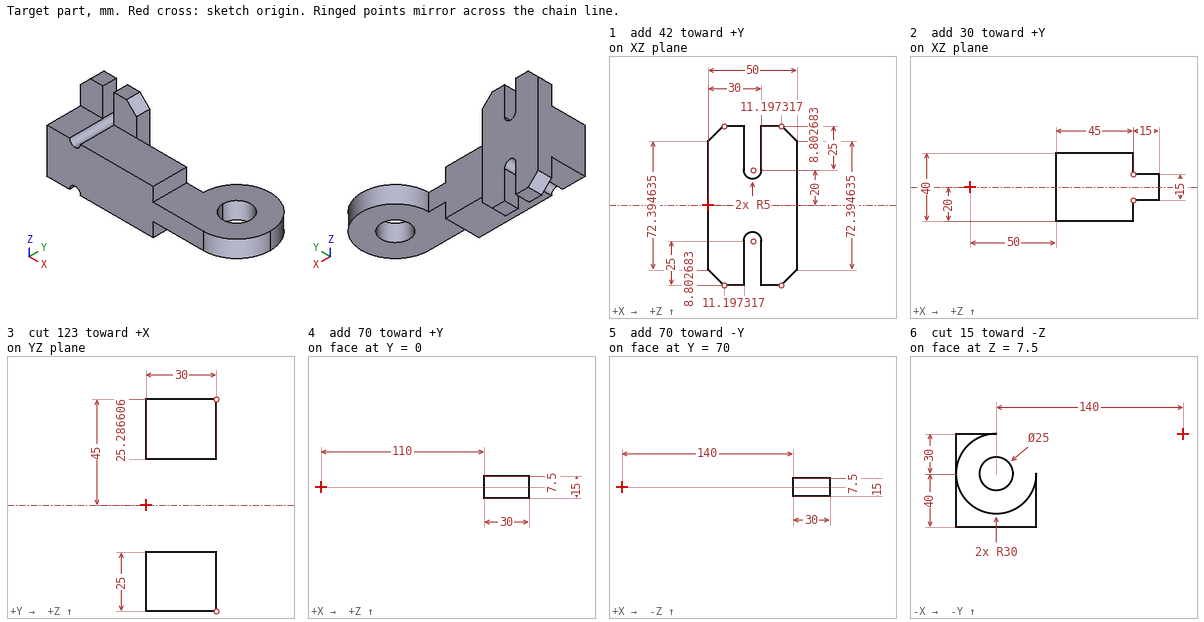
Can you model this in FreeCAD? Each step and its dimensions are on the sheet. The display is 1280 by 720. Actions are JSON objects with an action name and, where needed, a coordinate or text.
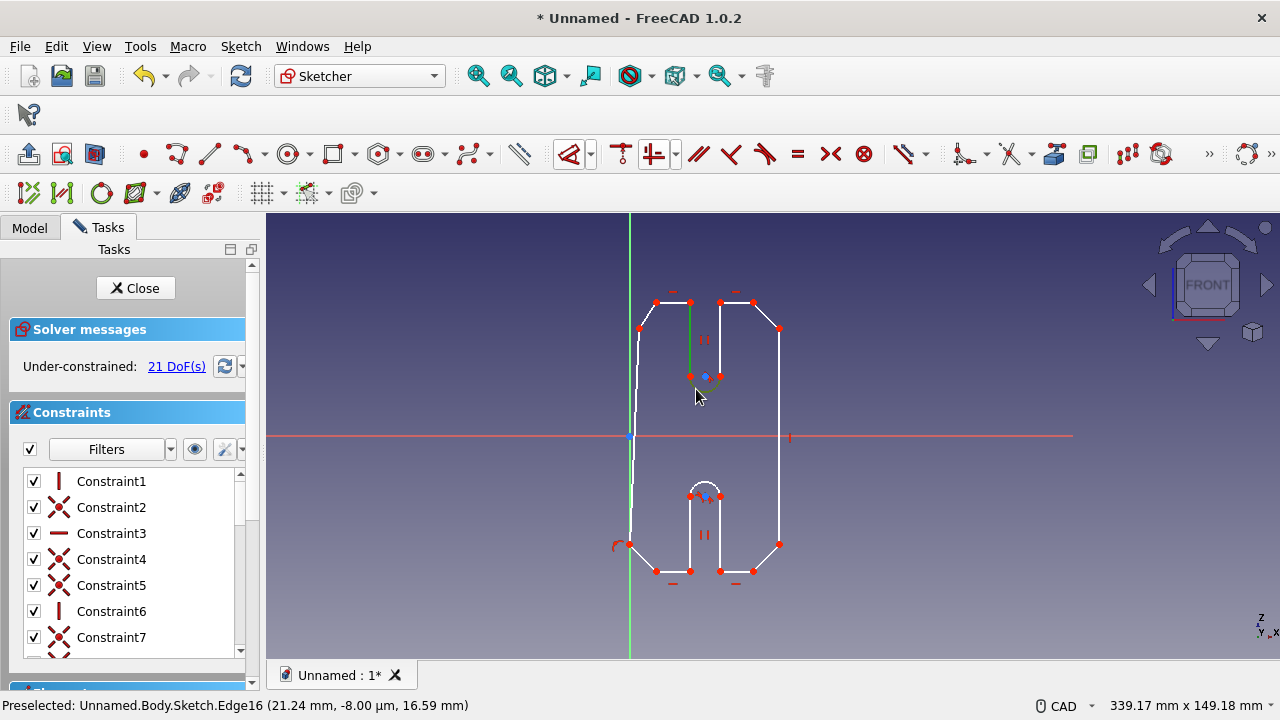
{"action": "left_click", "coordinate": [765, 154]}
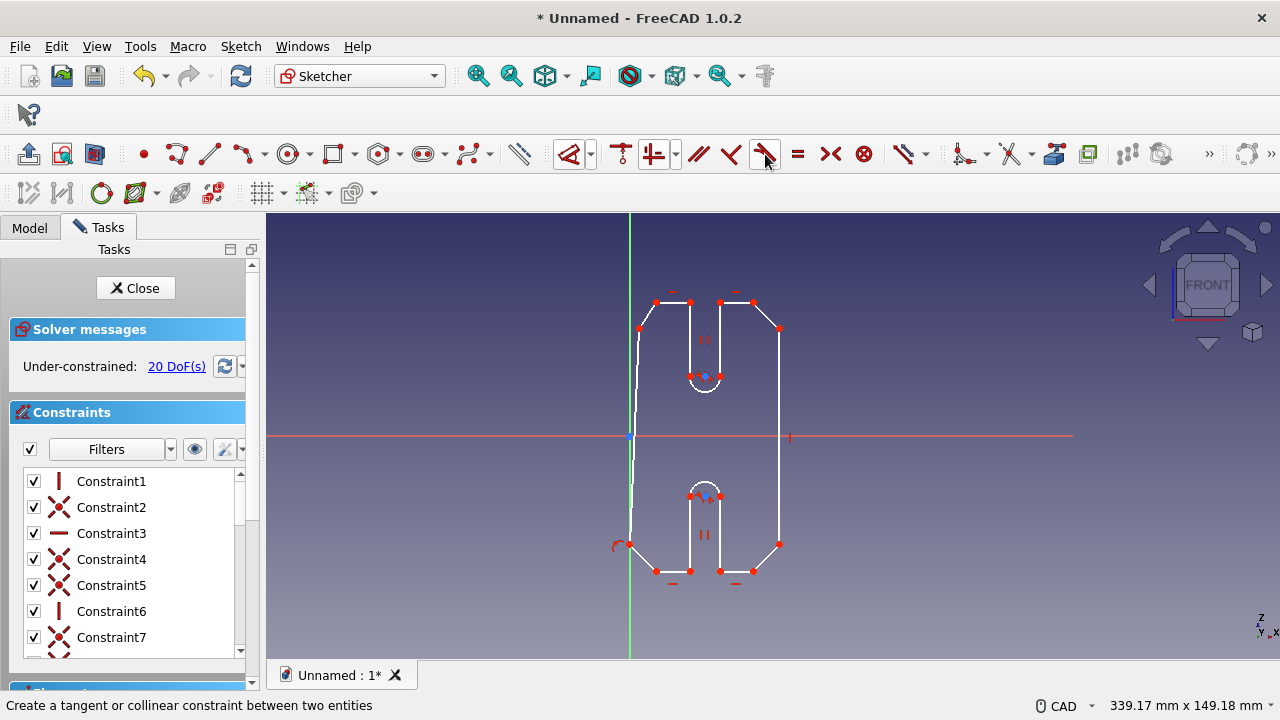
{"action": "left_click", "coordinate": [633, 480]}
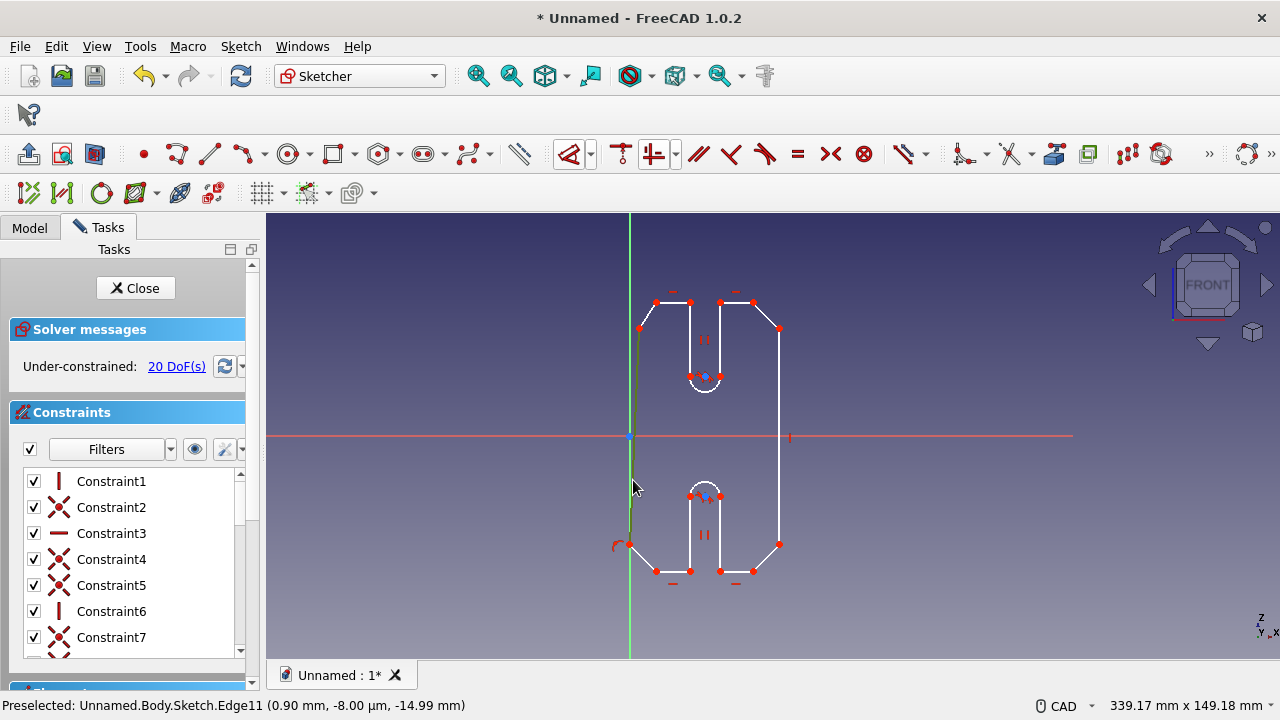
{"action": "left_click", "coordinate": [676, 154]}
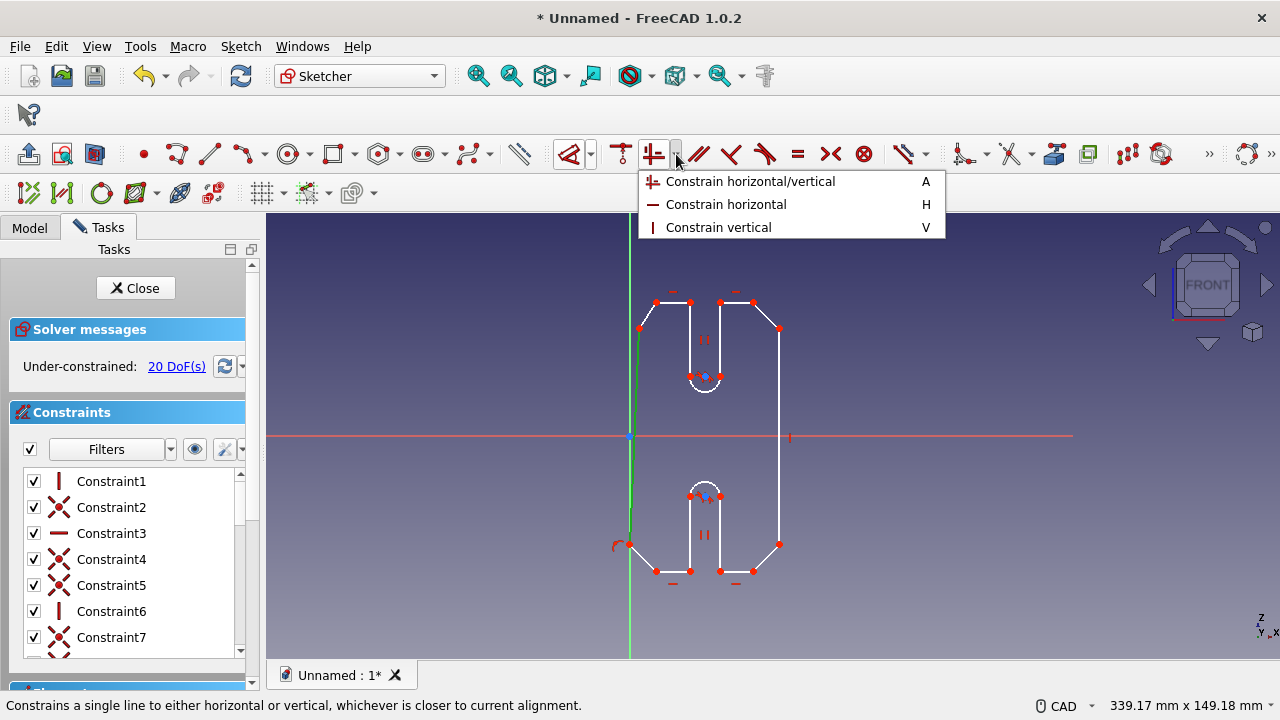
{"action": "left_click", "coordinate": [792, 228]}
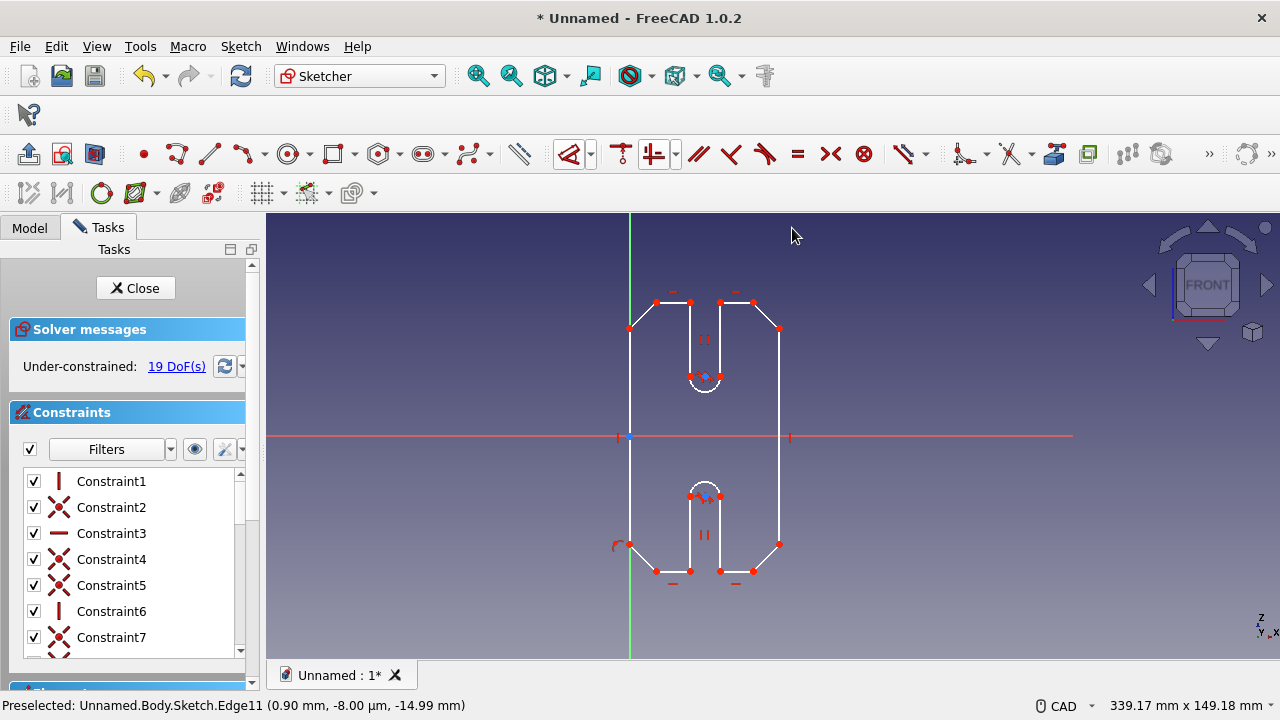
{"action": "left_click", "coordinate": [714, 485]}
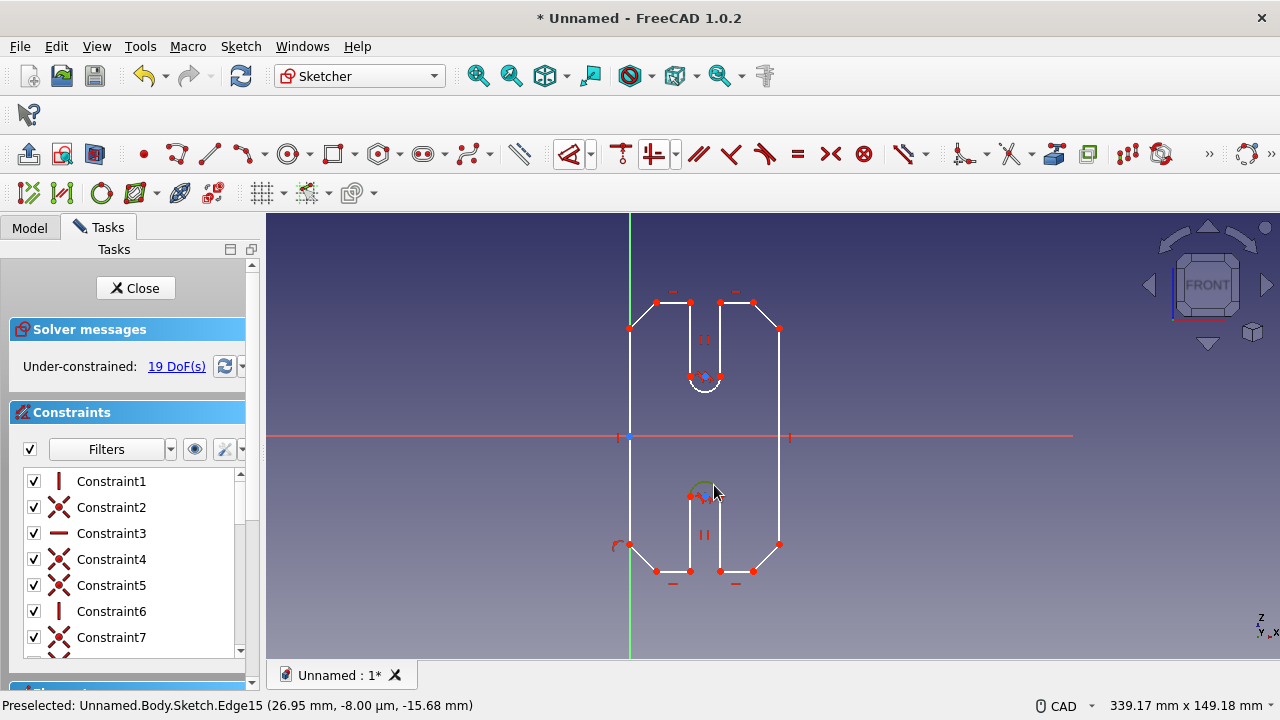
{"action": "left_click", "coordinate": [696, 389]}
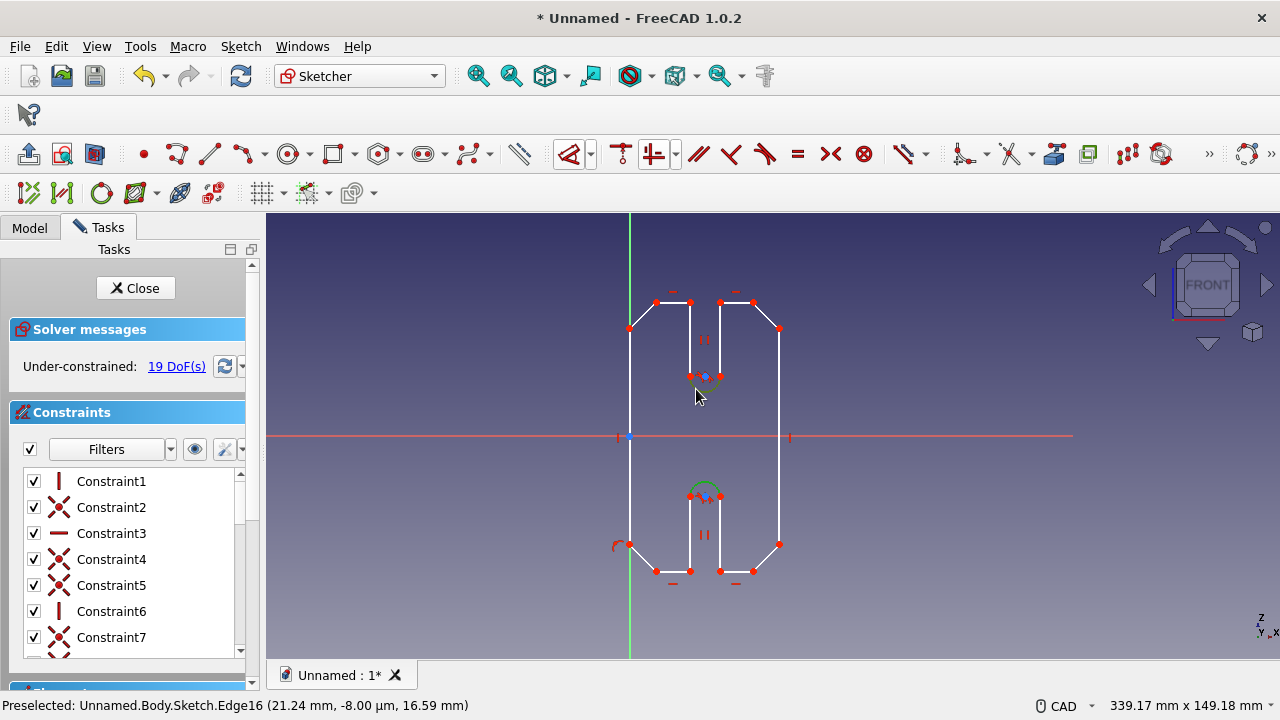
{"action": "left_click", "coordinate": [798, 154]}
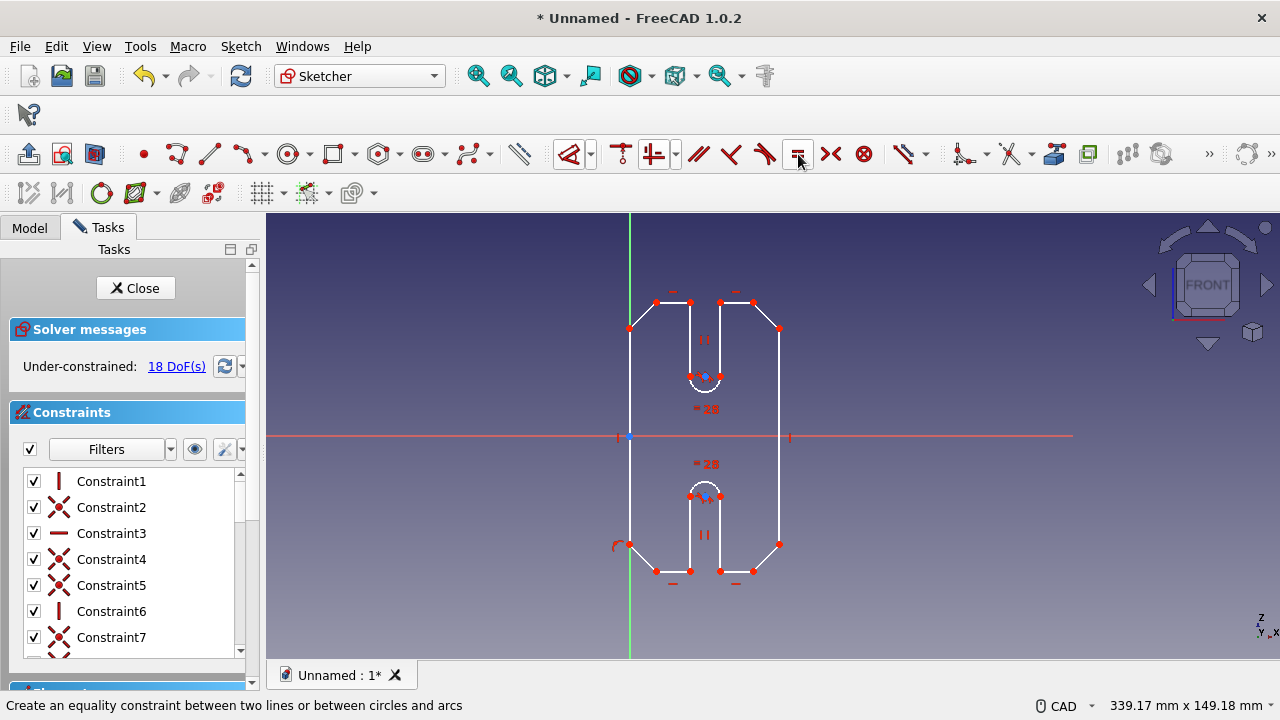
{"action": "left_click", "coordinate": [705, 497]}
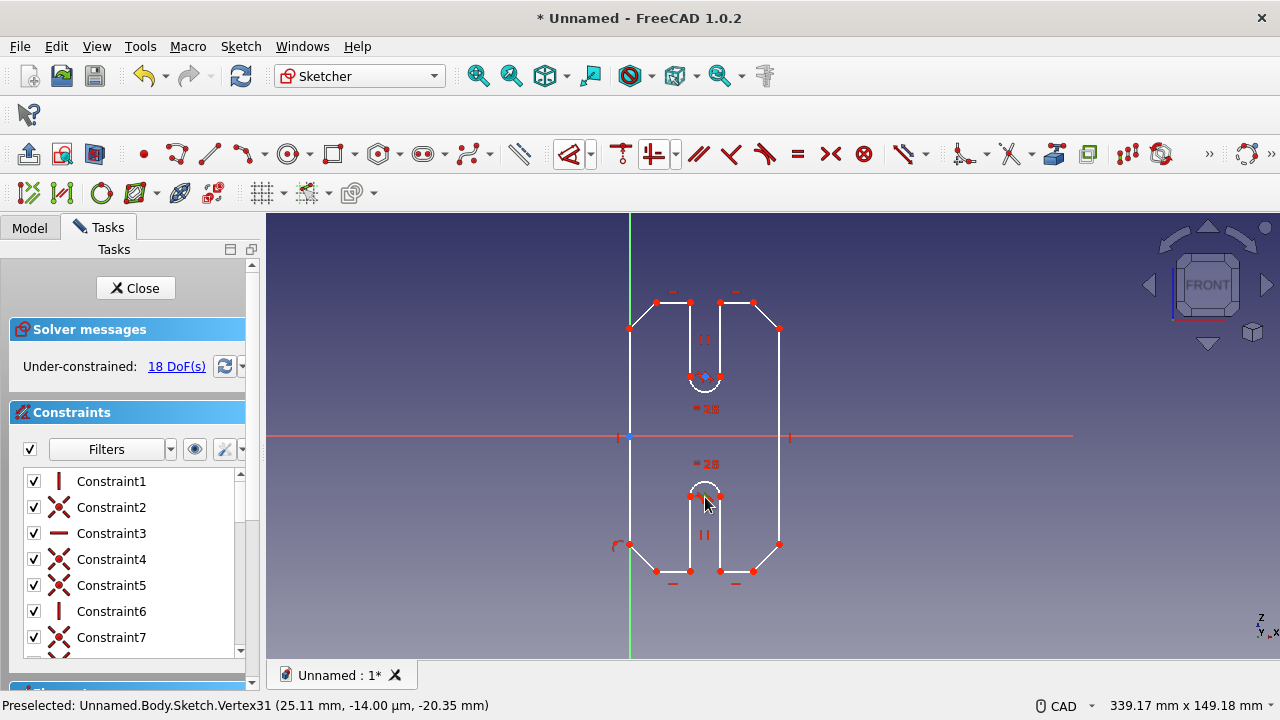
{"action": "left_click", "coordinate": [705, 377]}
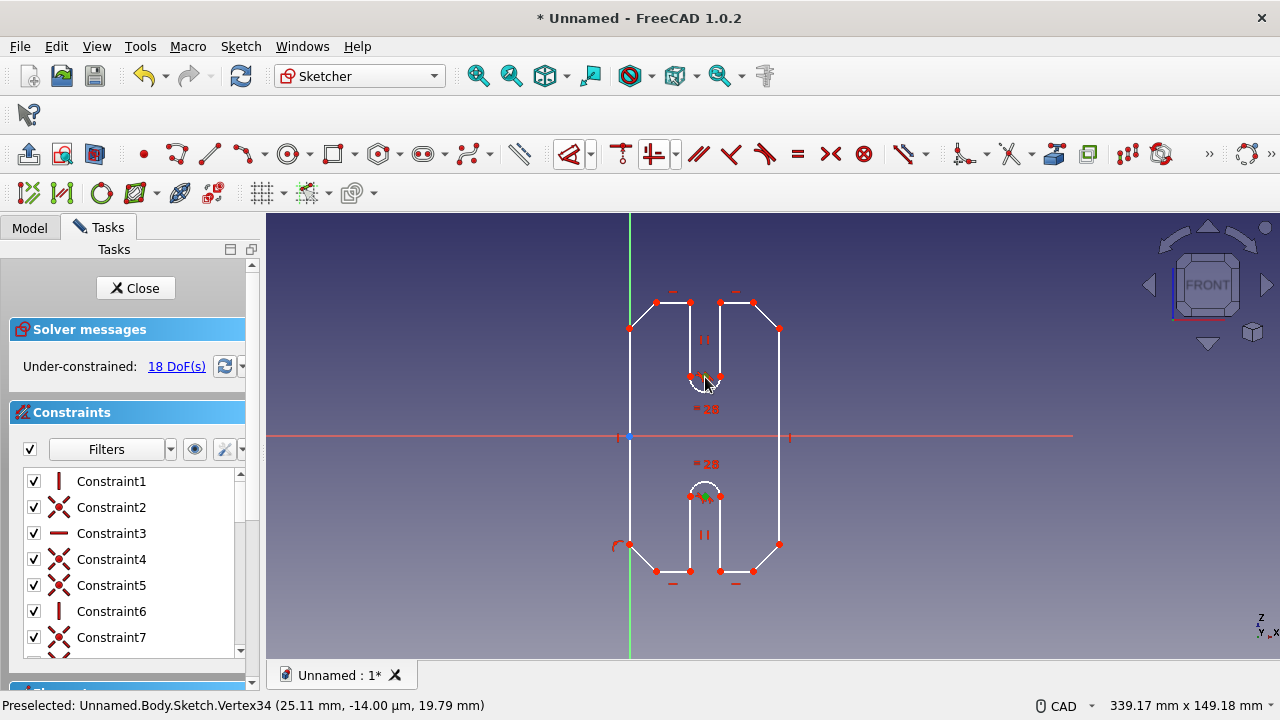
{"action": "left_click", "coordinate": [353, 436]}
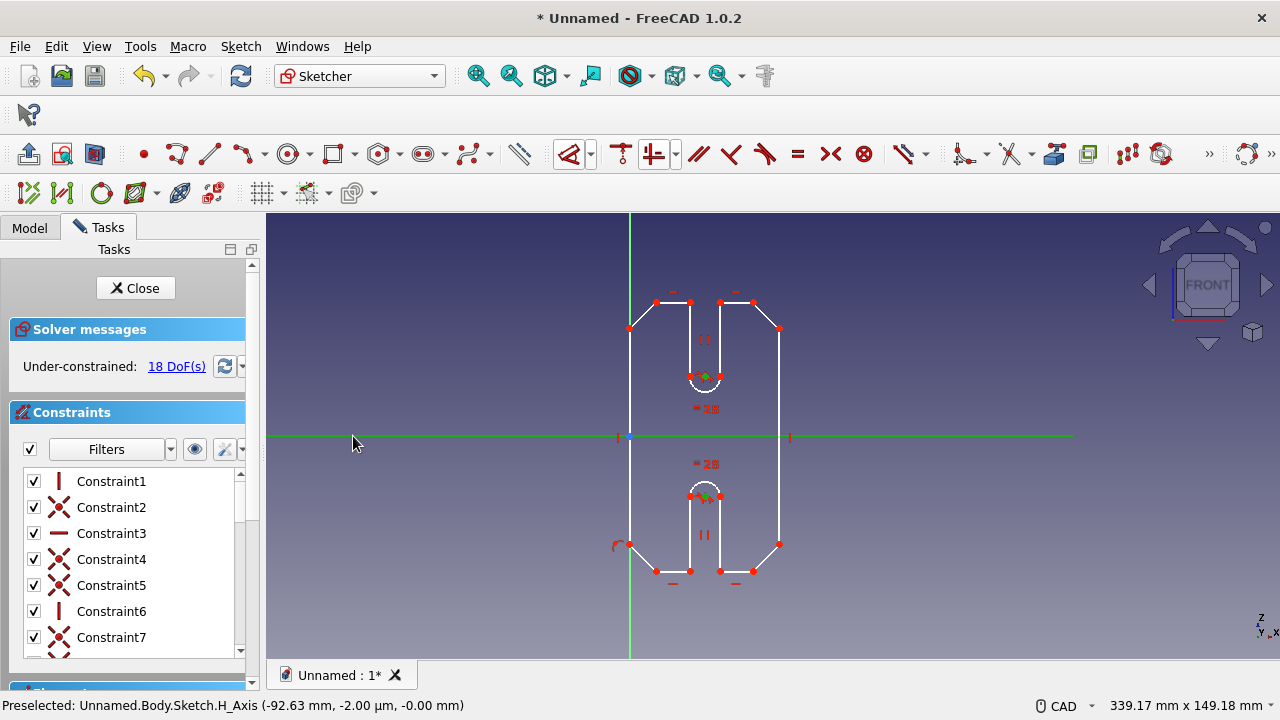
{"action": "key", "text": "s"}